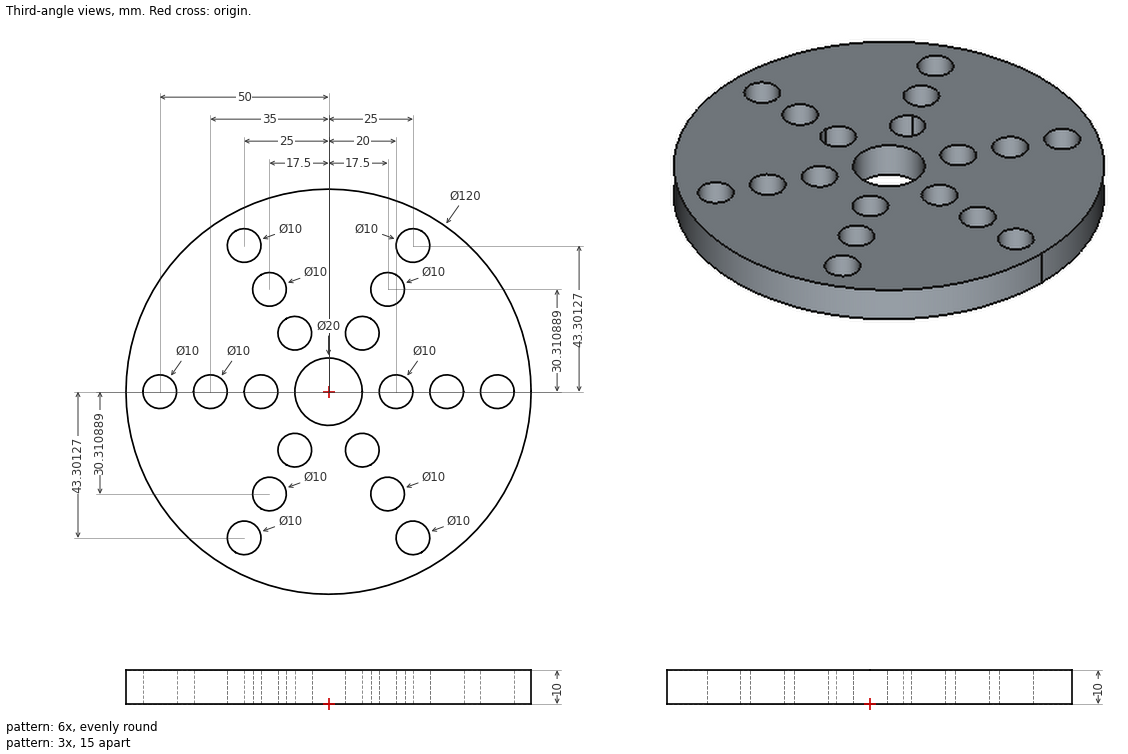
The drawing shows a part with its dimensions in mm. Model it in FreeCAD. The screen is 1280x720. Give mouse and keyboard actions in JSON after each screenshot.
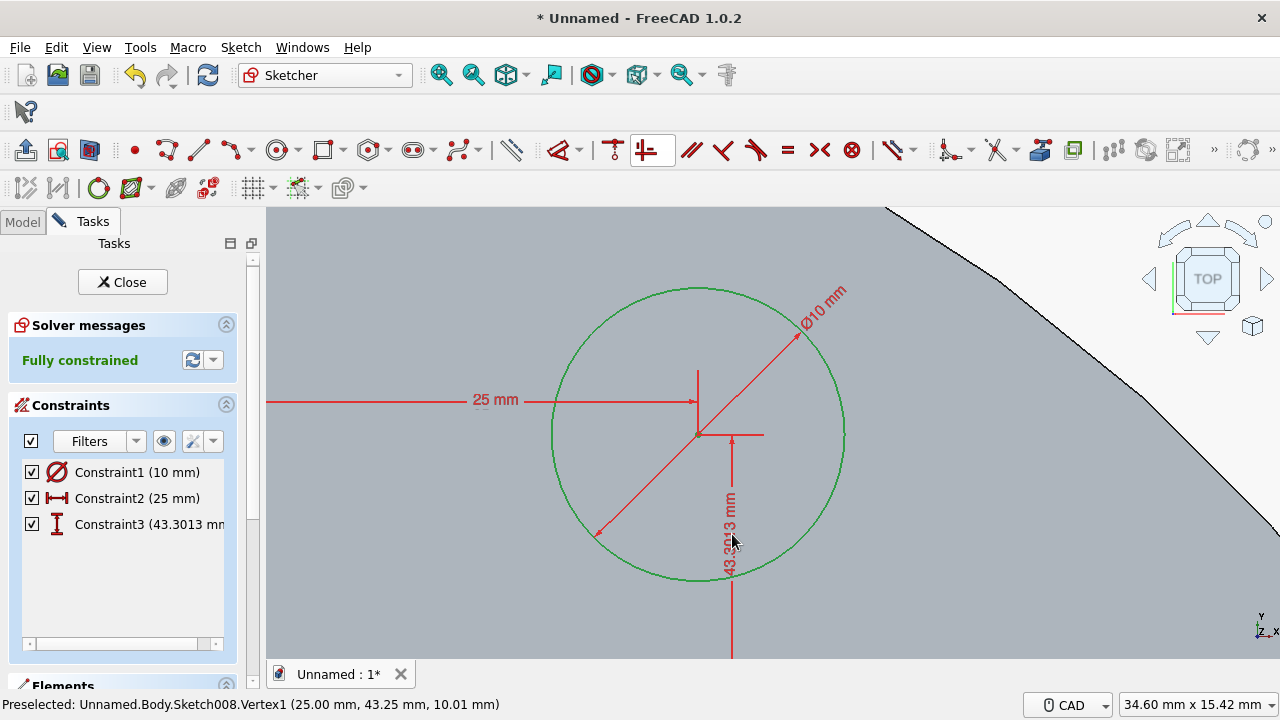
{"action": "left_click", "coordinate": [123, 282]}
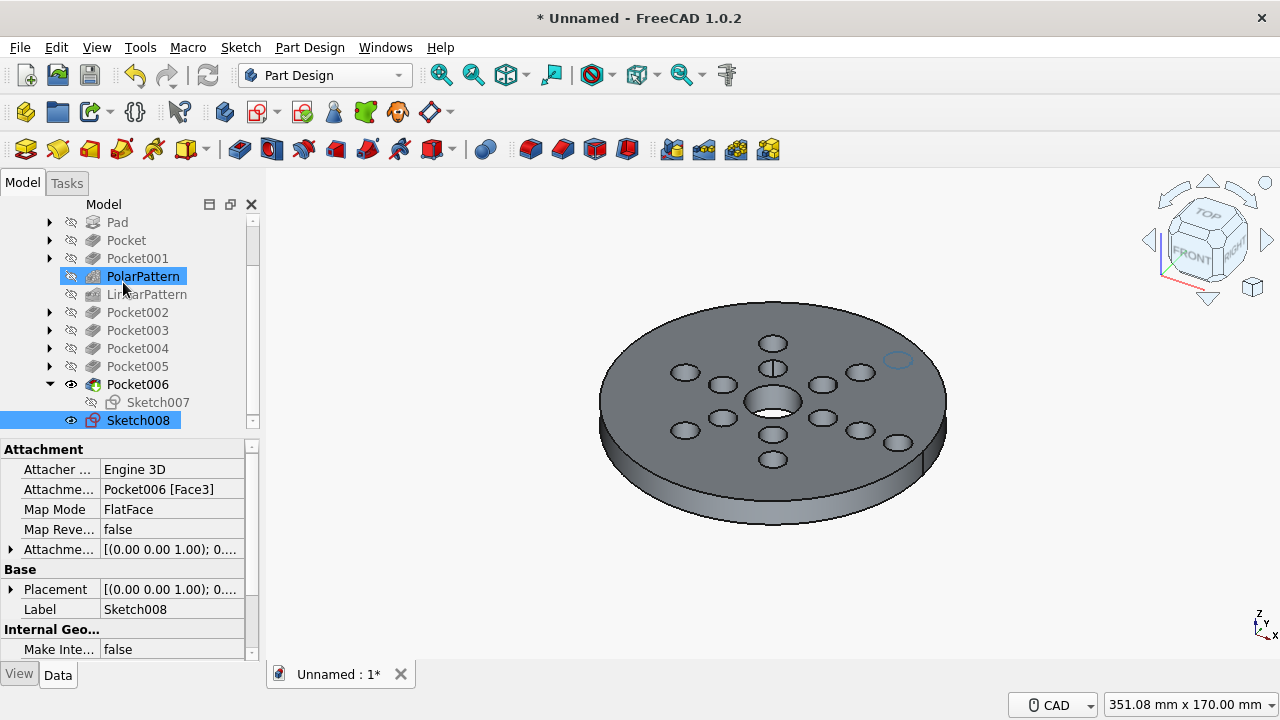
{"action": "left_click", "coordinate": [240, 150]}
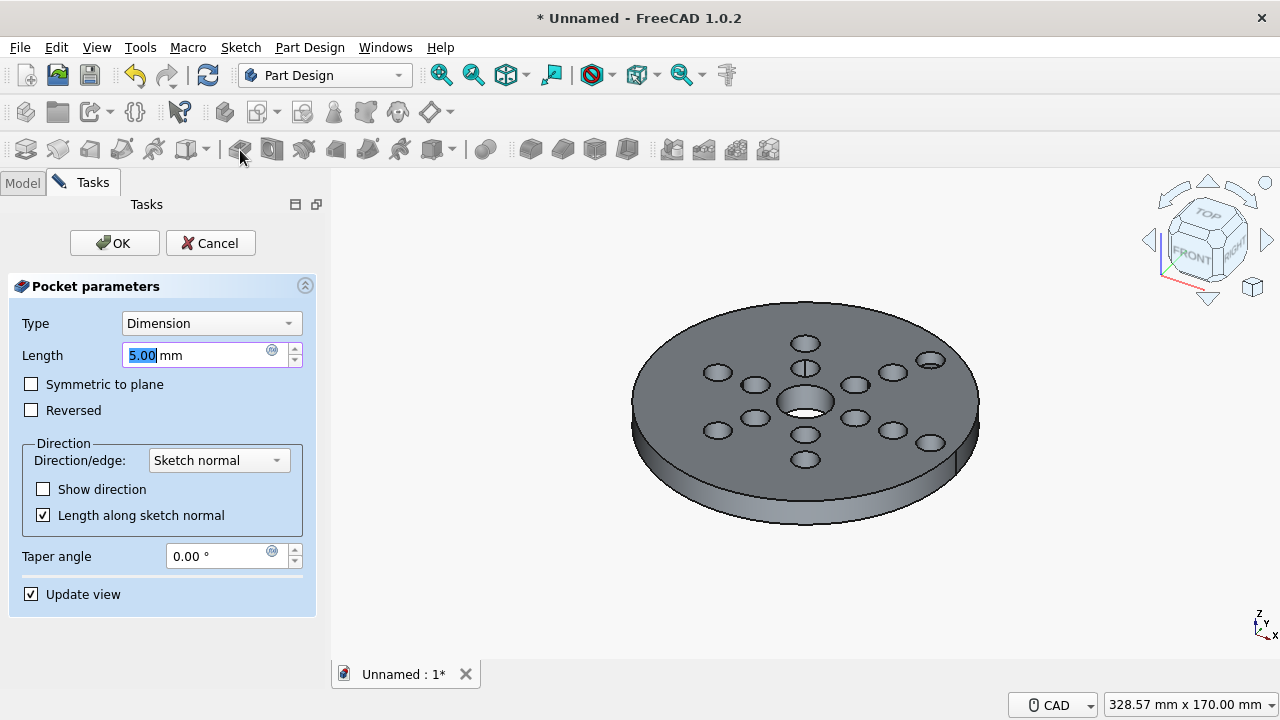
{"action": "type", "text": "10"}
{"action": "key", "text": "Tab"}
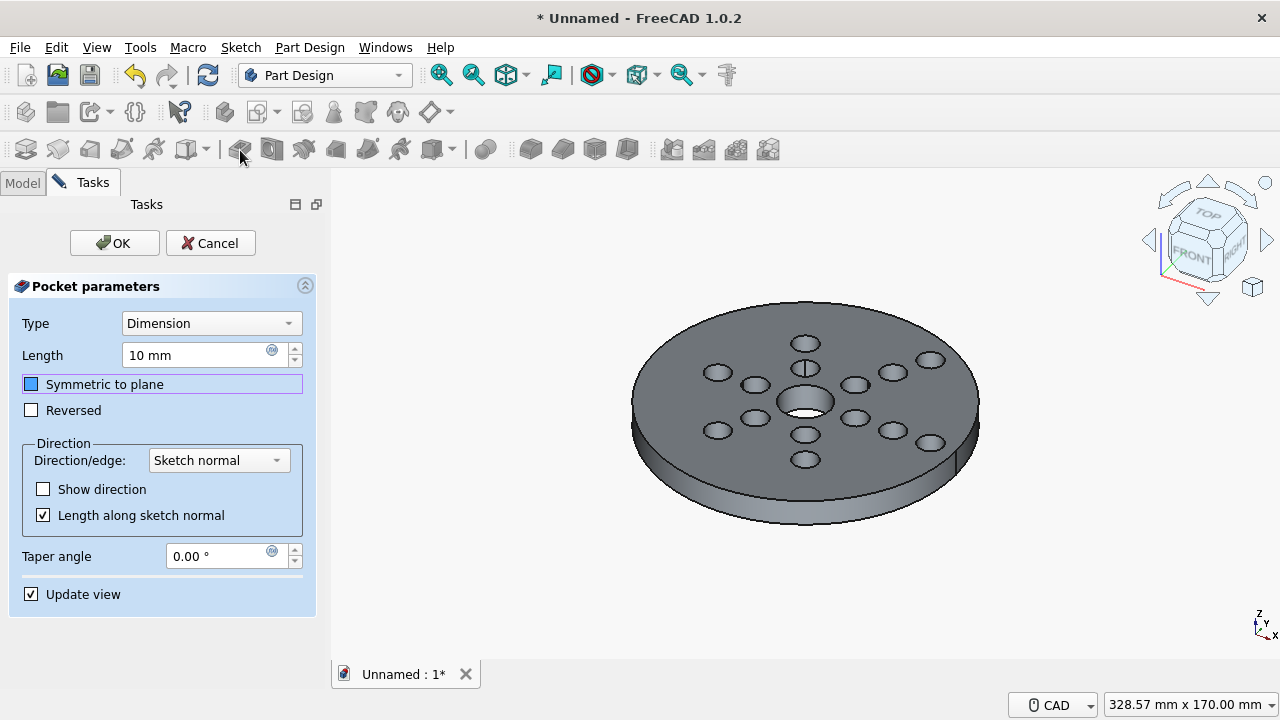
{"action": "left_click", "coordinate": [115, 243]}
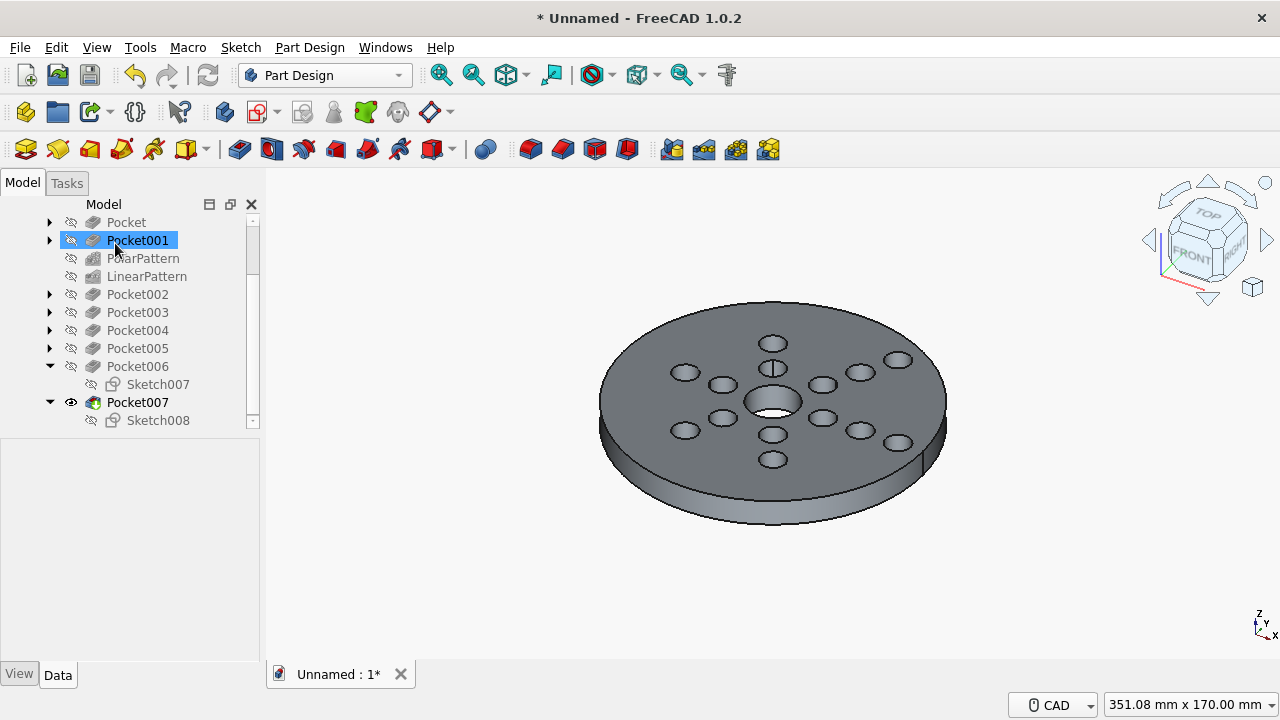
{"action": "left_click", "coordinate": [823, 351]}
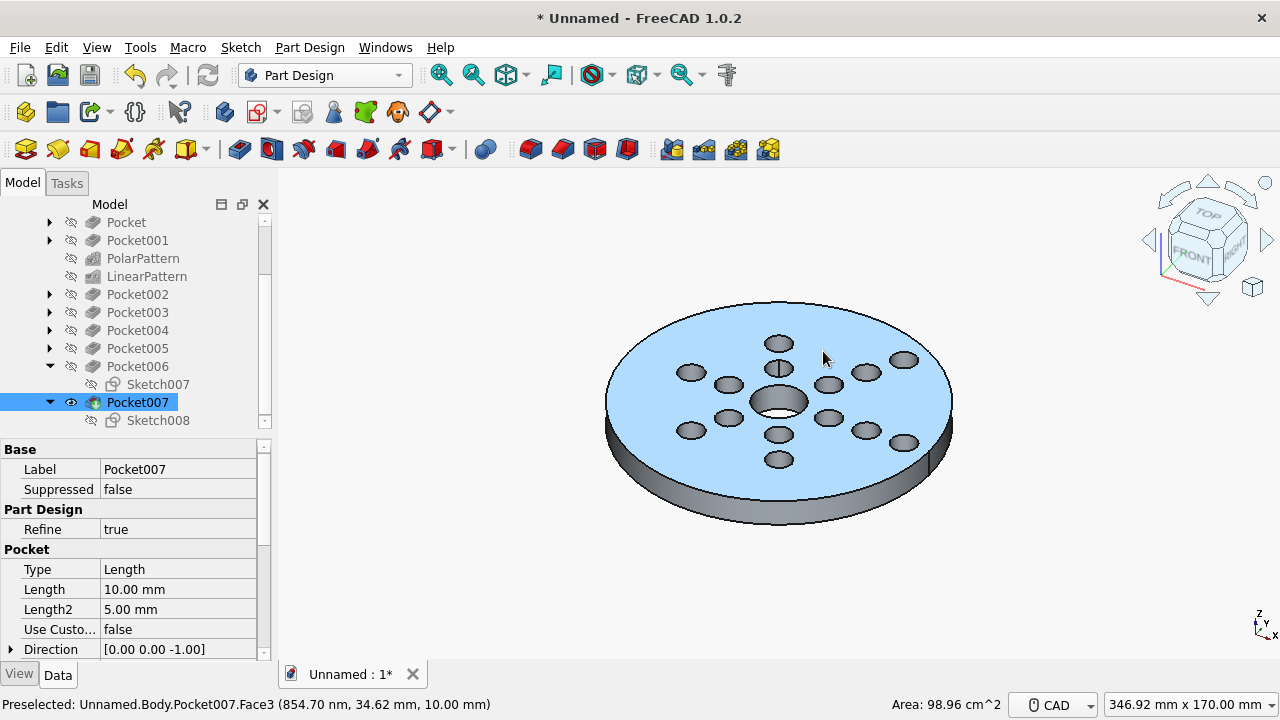
{"action": "left_click", "coordinate": [258, 112]}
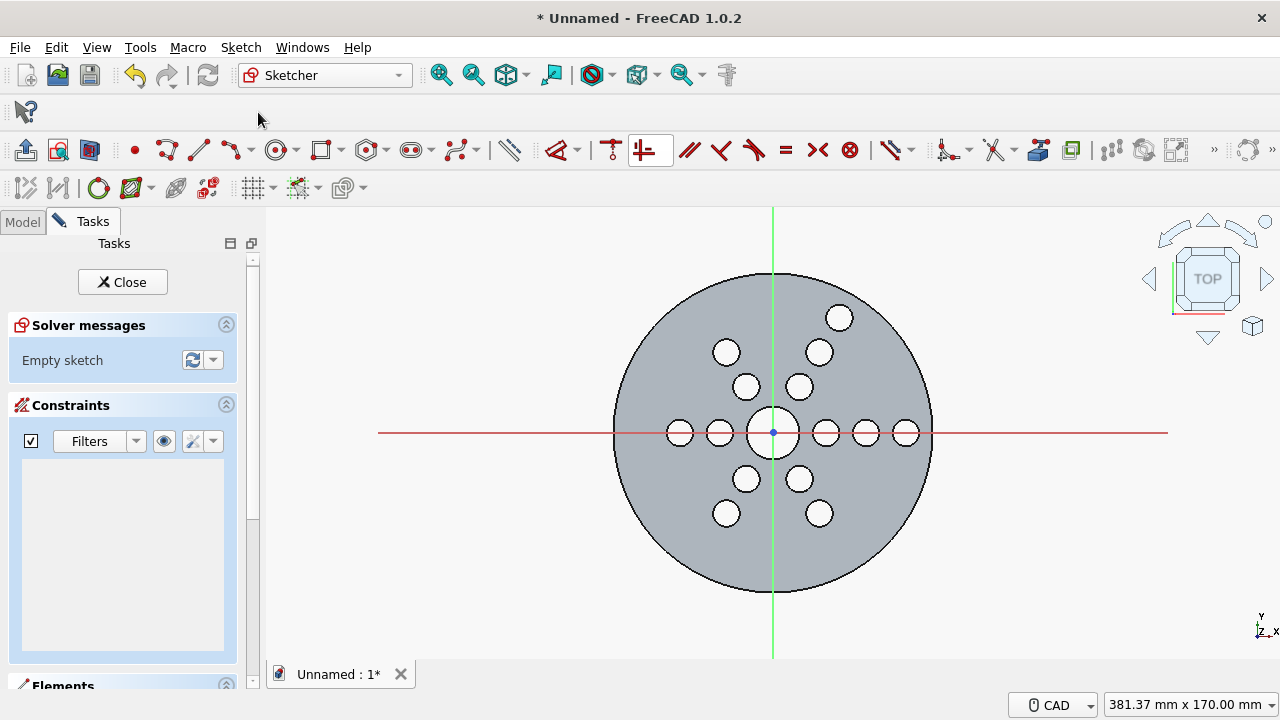
{"action": "scroll", "coordinate": [707, 306], "scroll_direction": "up", "scroll_amount": 12}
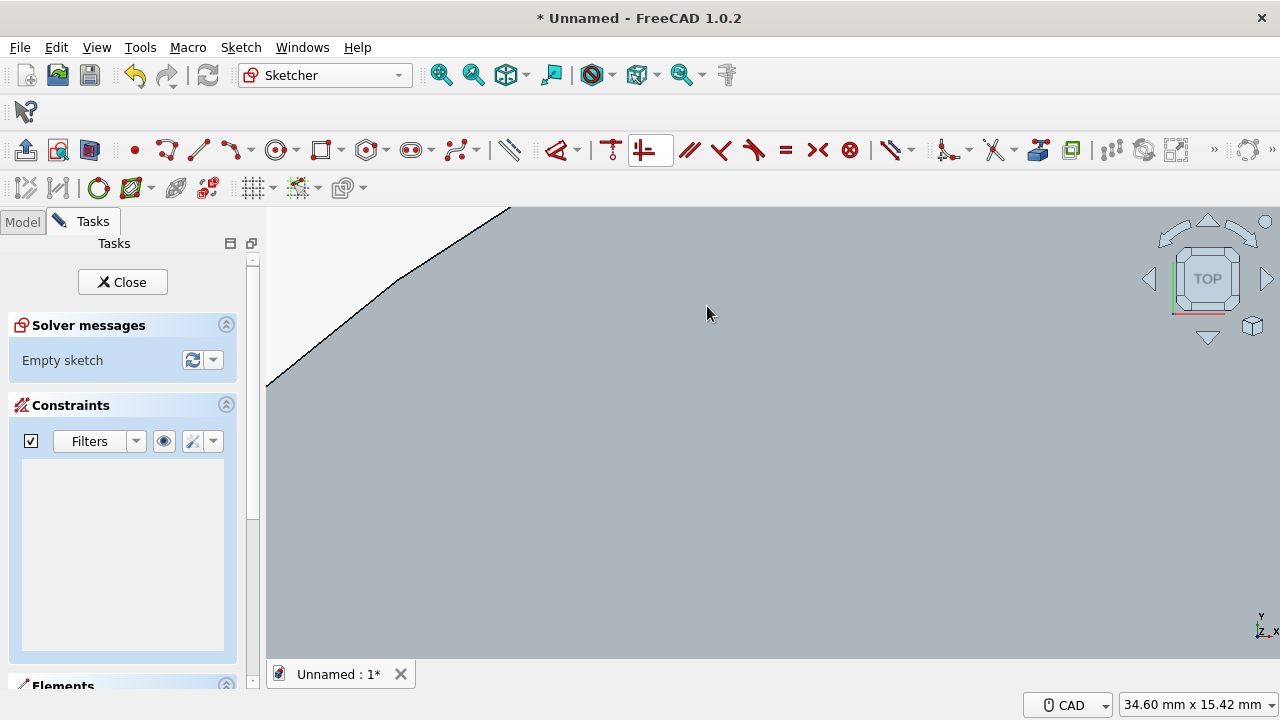
{"action": "left_click", "coordinate": [276, 150]}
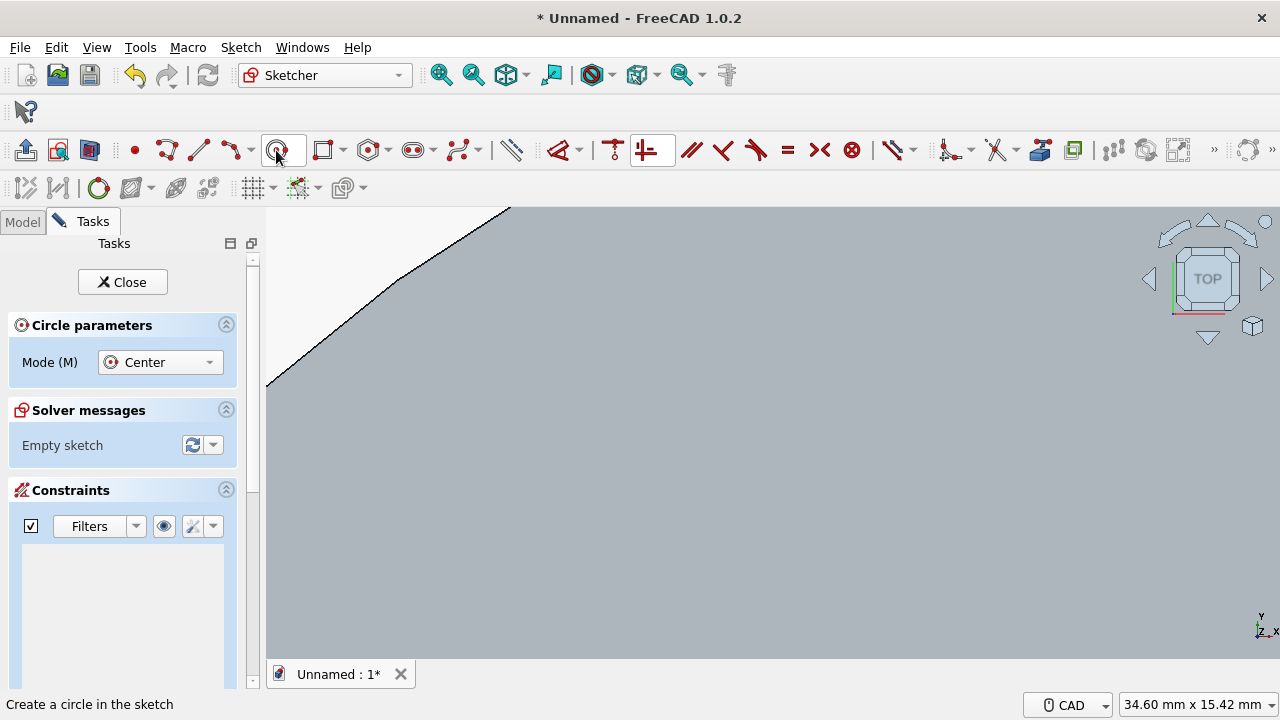
{"action": "left_click", "coordinate": [697, 435]}
{"action": "left_click", "coordinate": [801, 331]}
{"action": "key", "text": "Escape"}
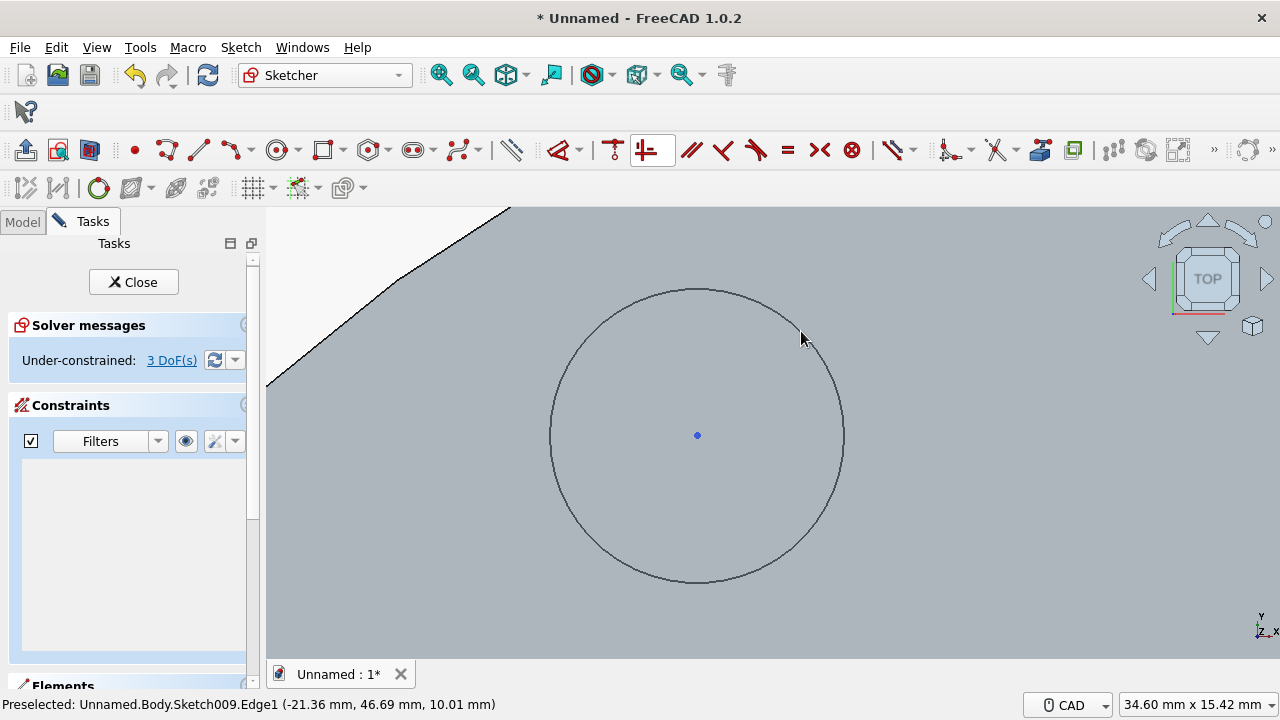
{"action": "left_click", "coordinate": [558, 150]}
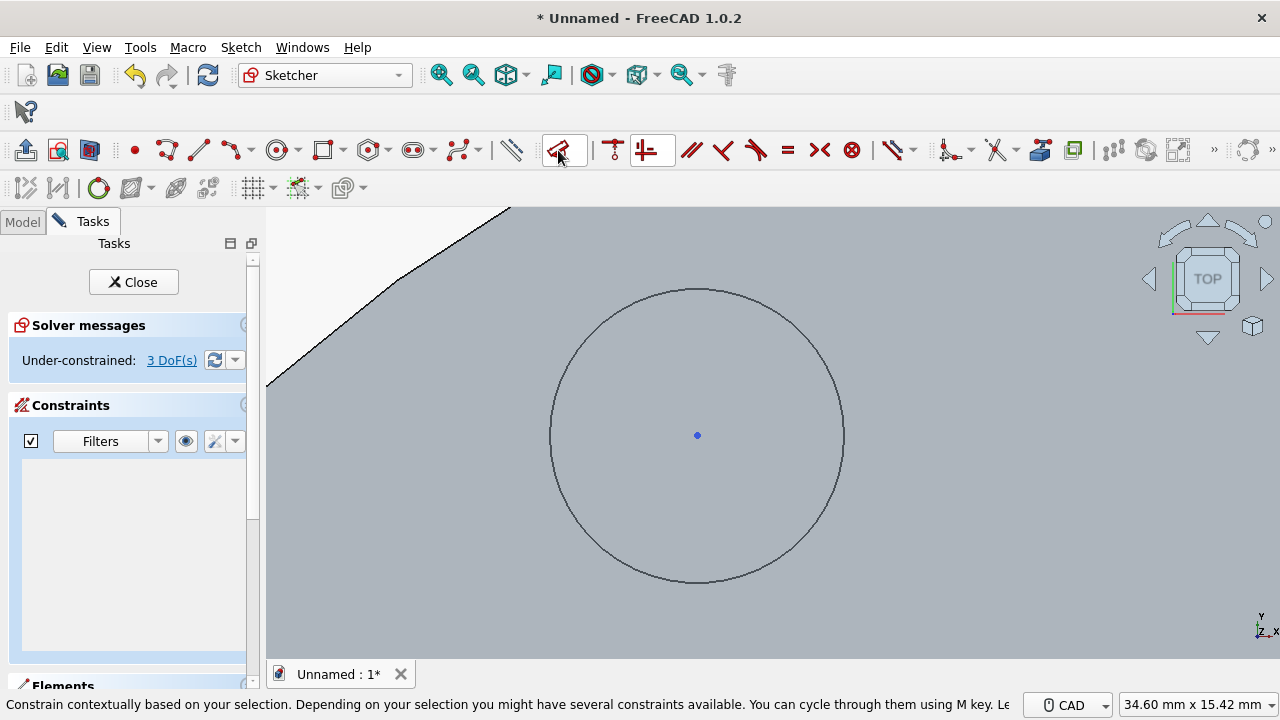
{"action": "left_click", "coordinate": [801, 332]}
{"action": "left_click", "coordinate": [824, 309]}